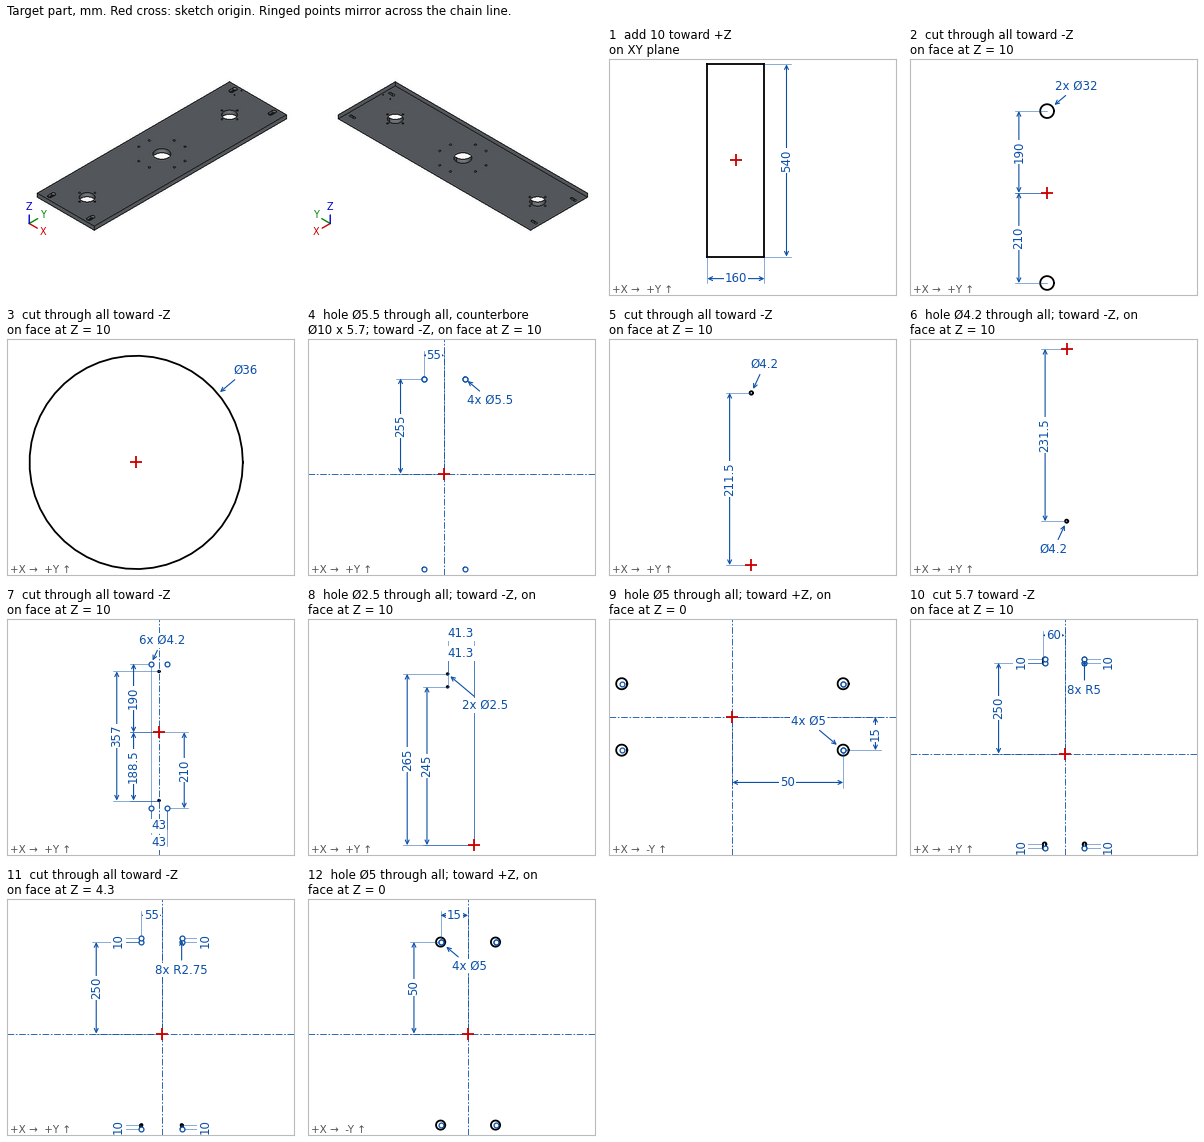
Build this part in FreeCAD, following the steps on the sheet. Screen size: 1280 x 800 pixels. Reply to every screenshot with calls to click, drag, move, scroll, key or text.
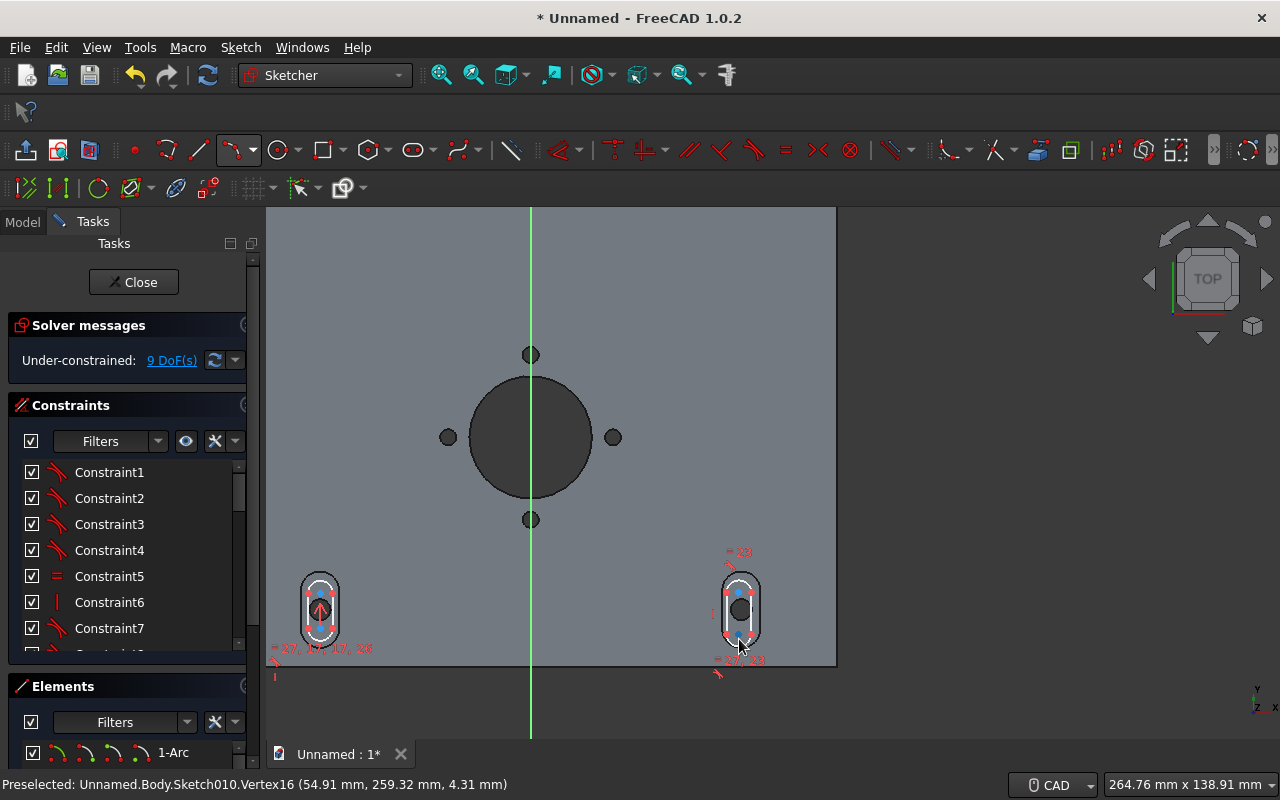
click(739, 634)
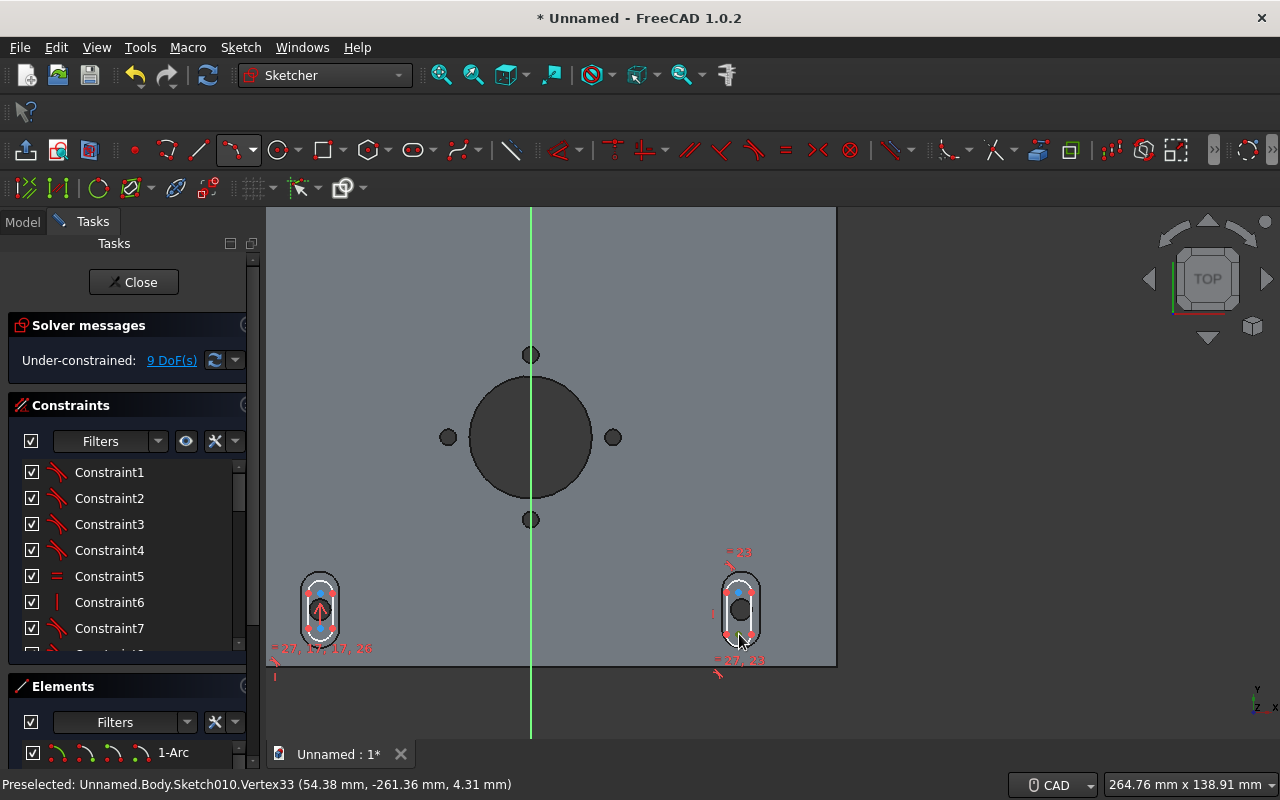
scroll(739, 639, down, 9)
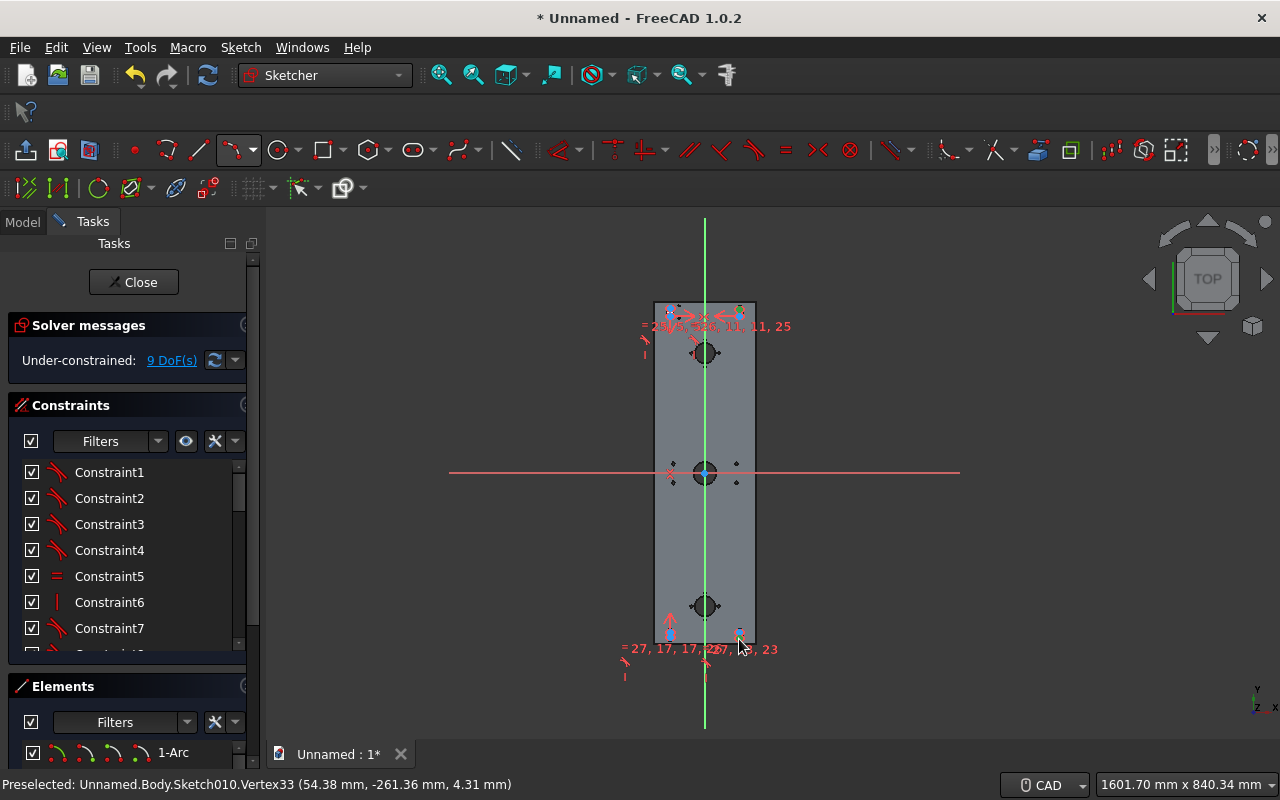
click(470, 473)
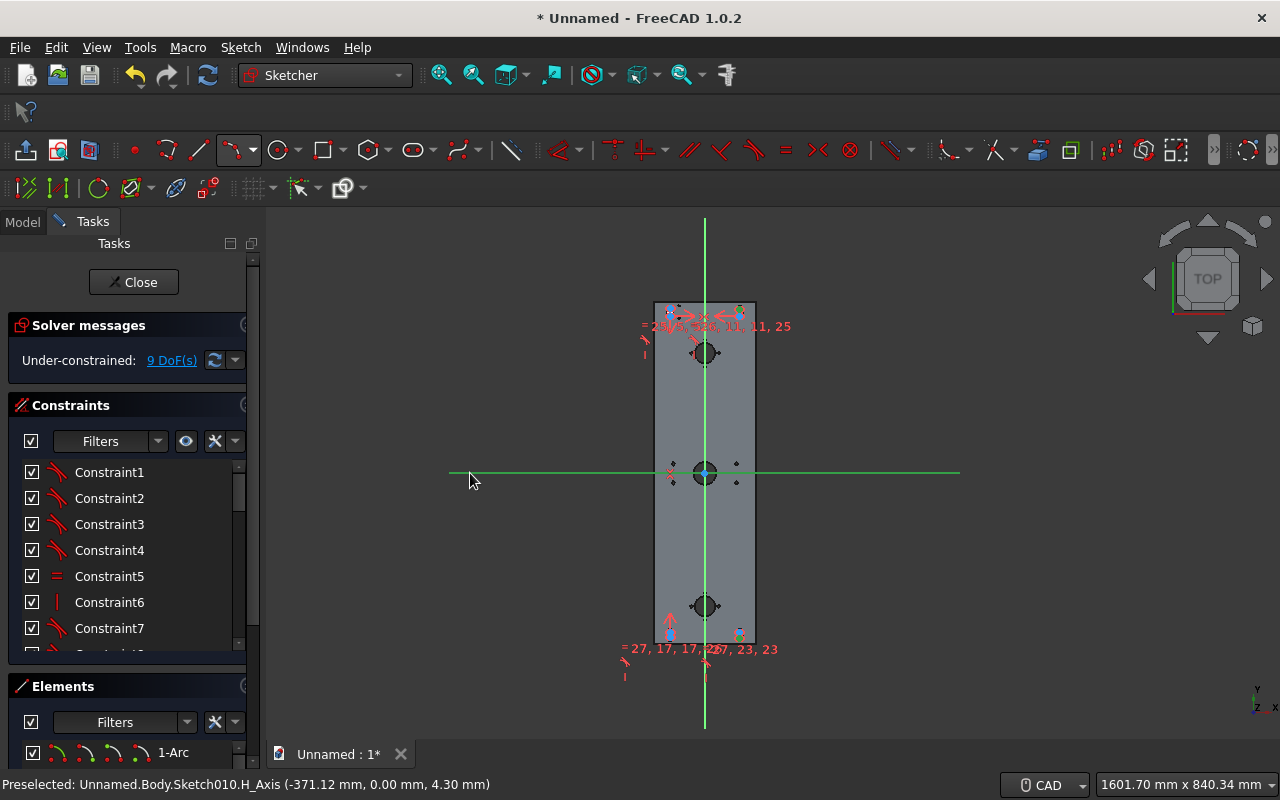
key(s)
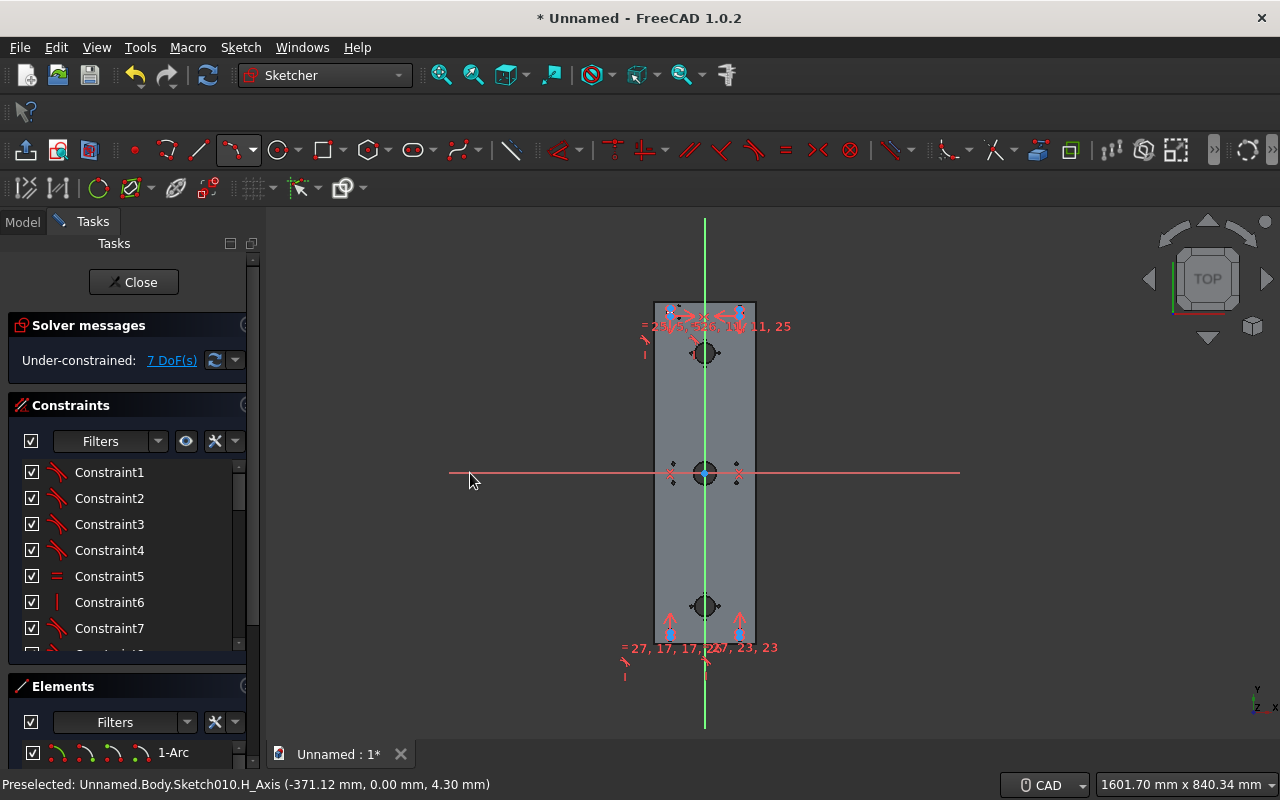
key(d)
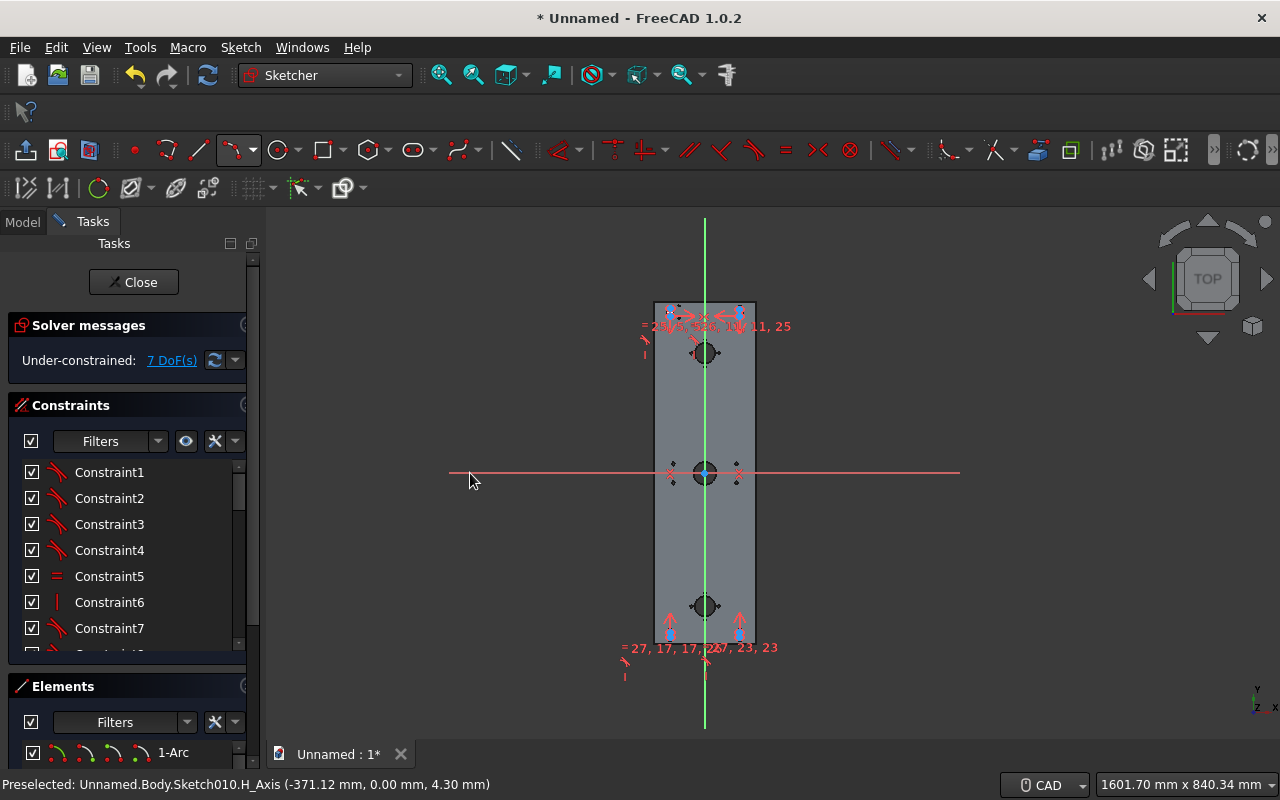
scroll(670, 318, up, 16)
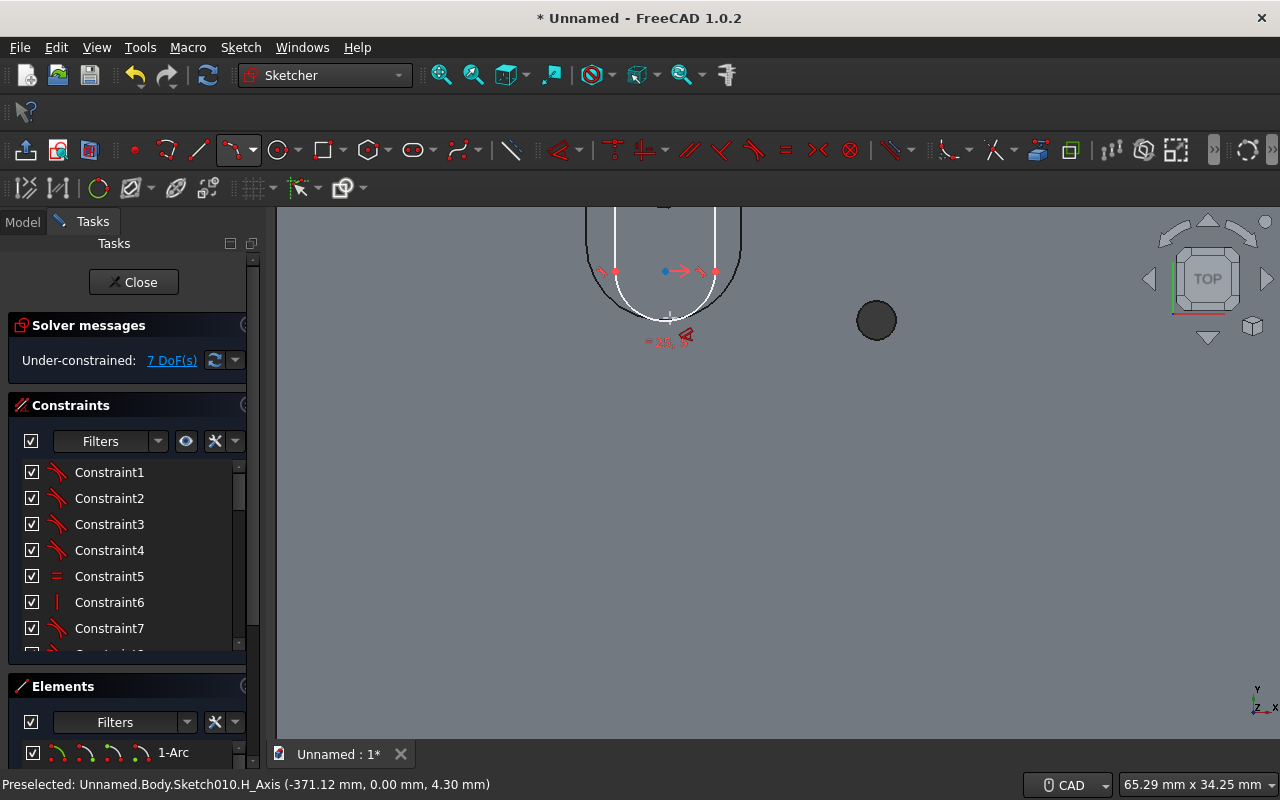
click(665, 321)
click(665, 353)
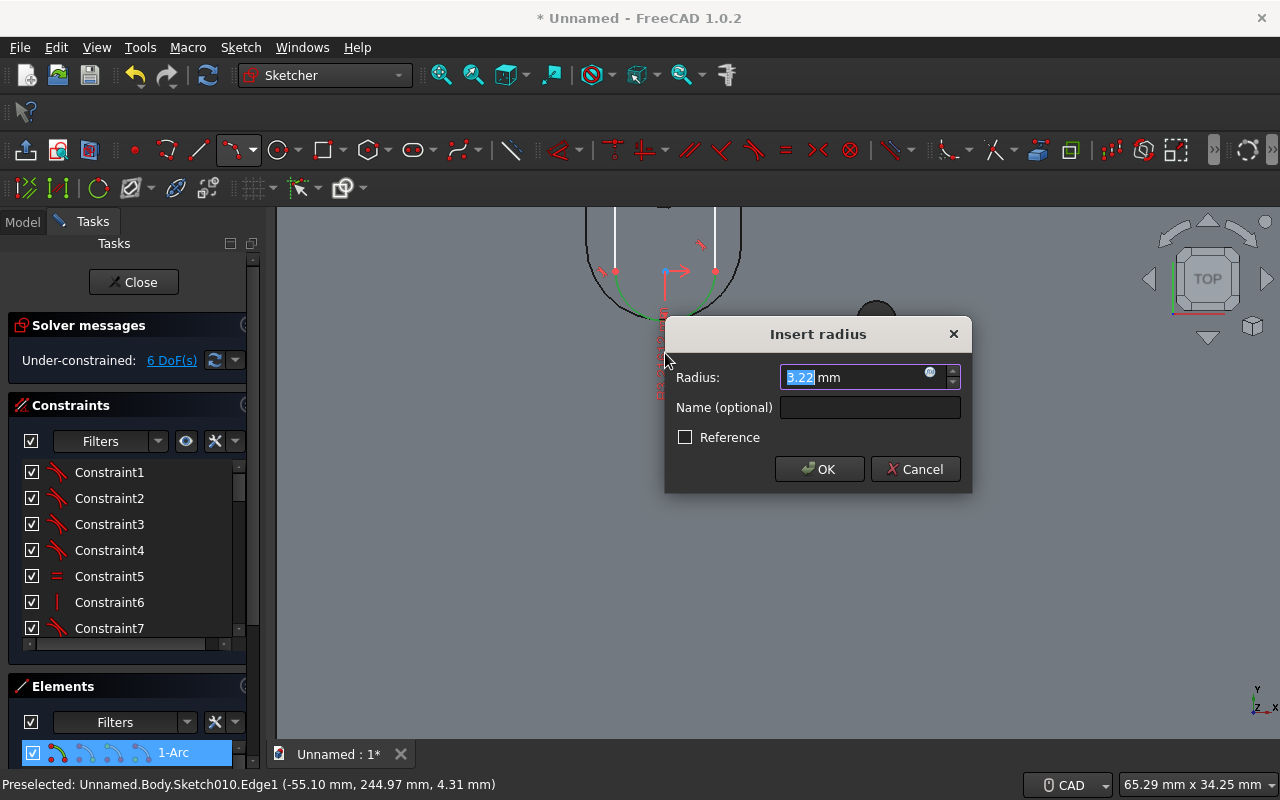
text(2.75)
key(Return)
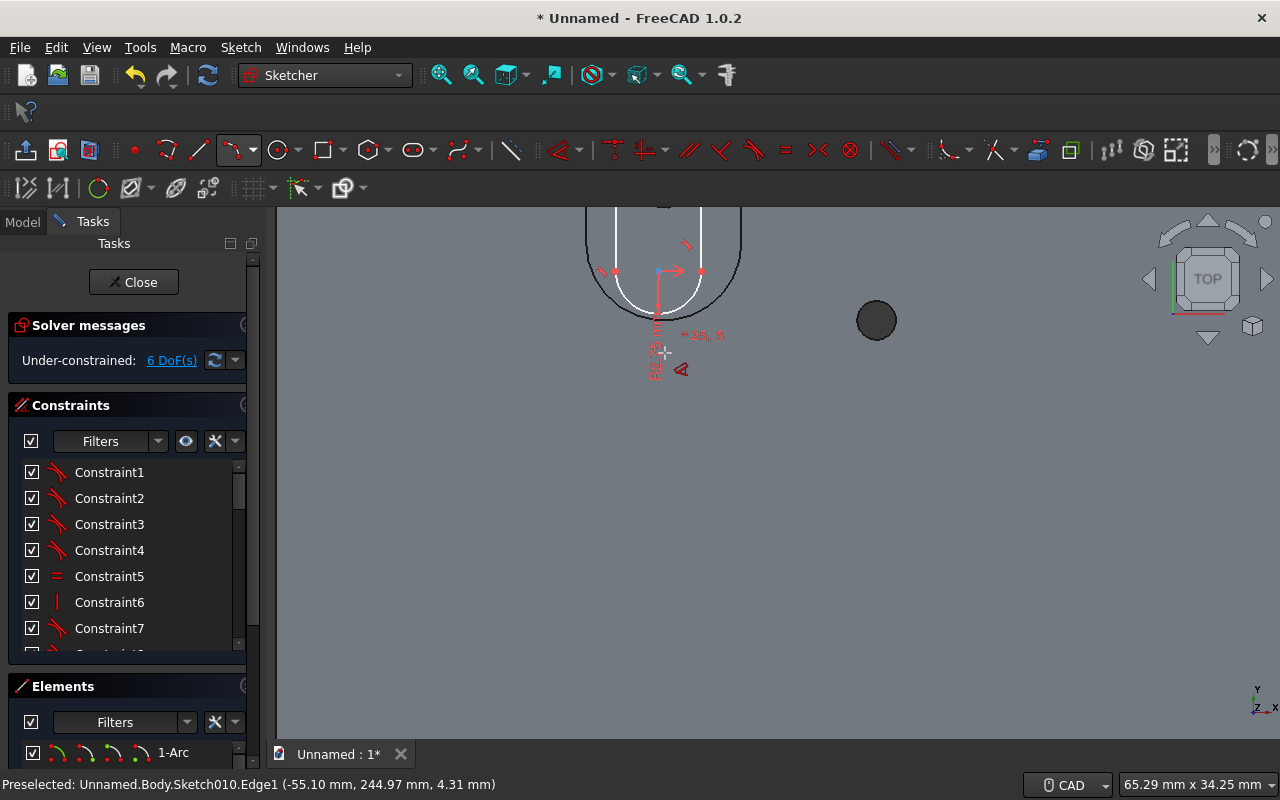
scroll(662, 282, down, 15)